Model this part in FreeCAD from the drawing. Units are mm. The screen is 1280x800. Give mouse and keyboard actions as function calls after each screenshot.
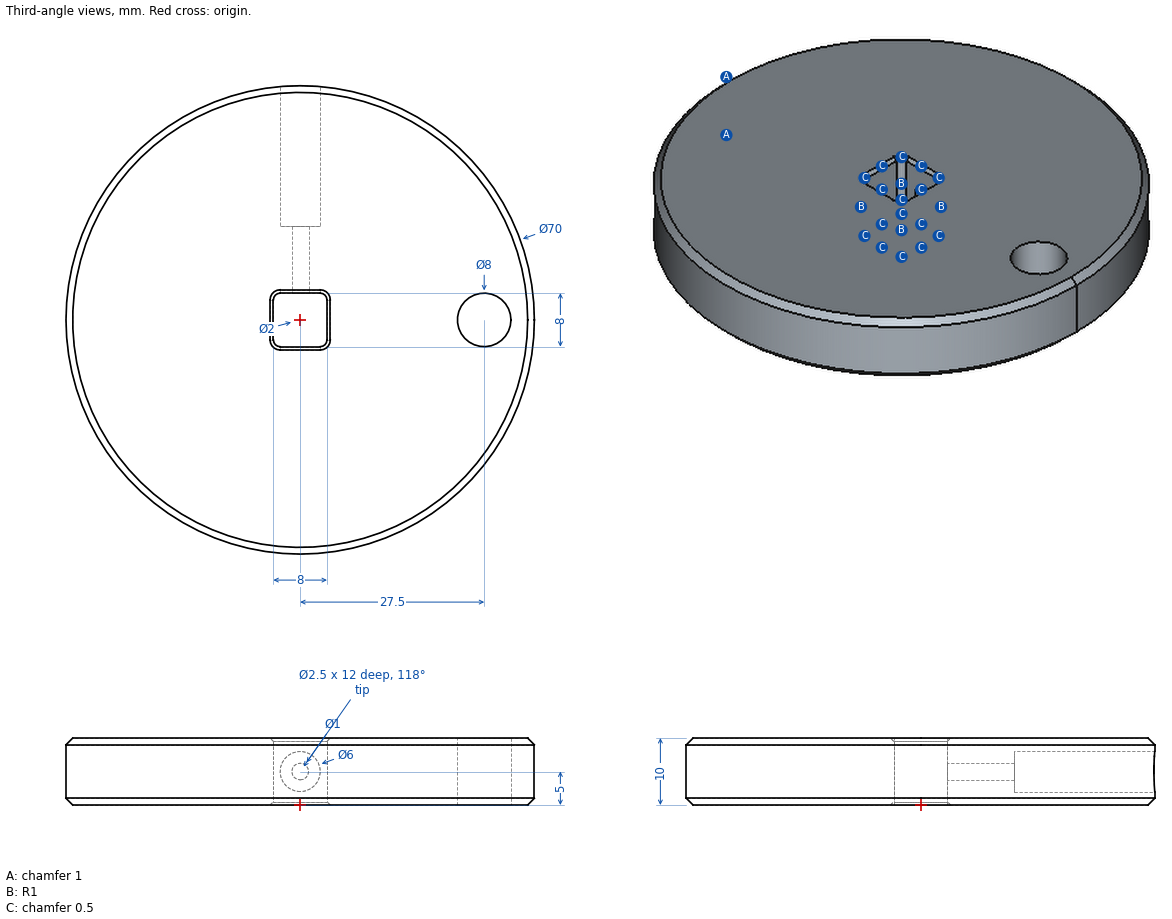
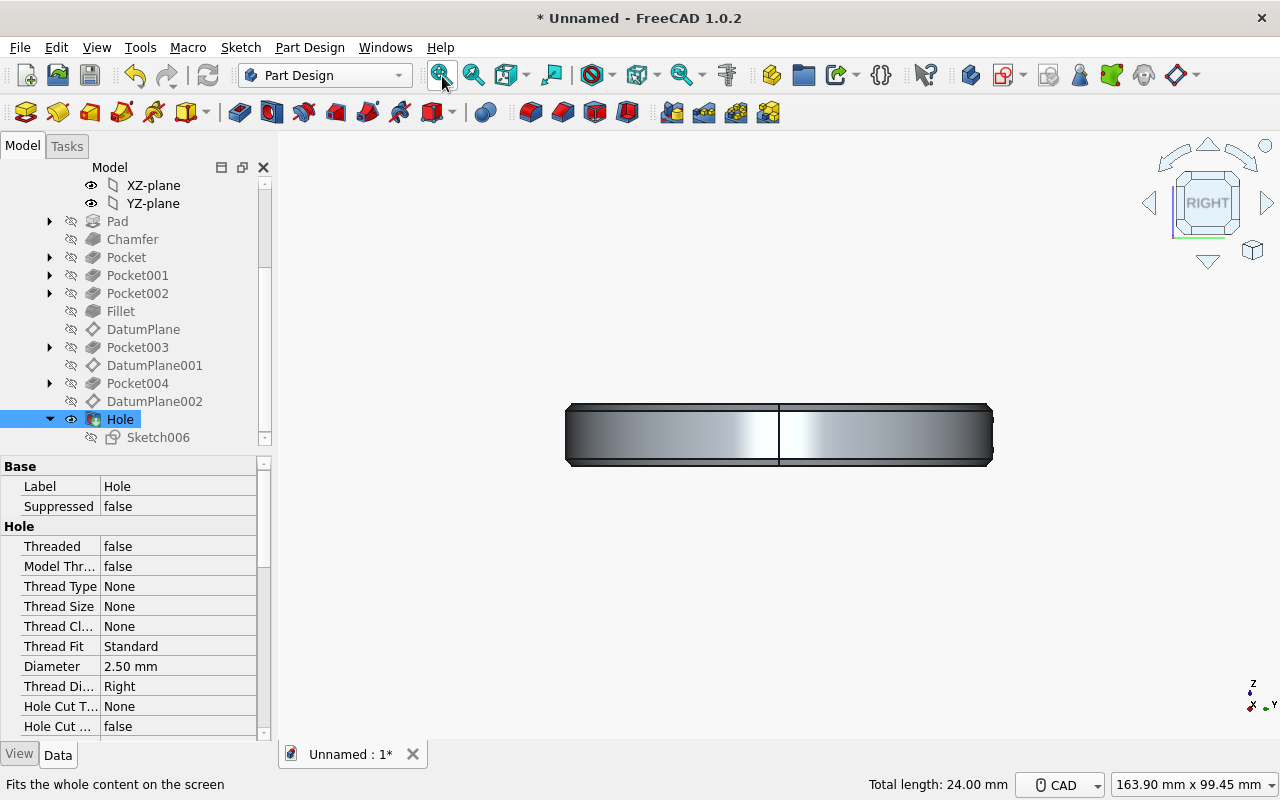
click(442, 76)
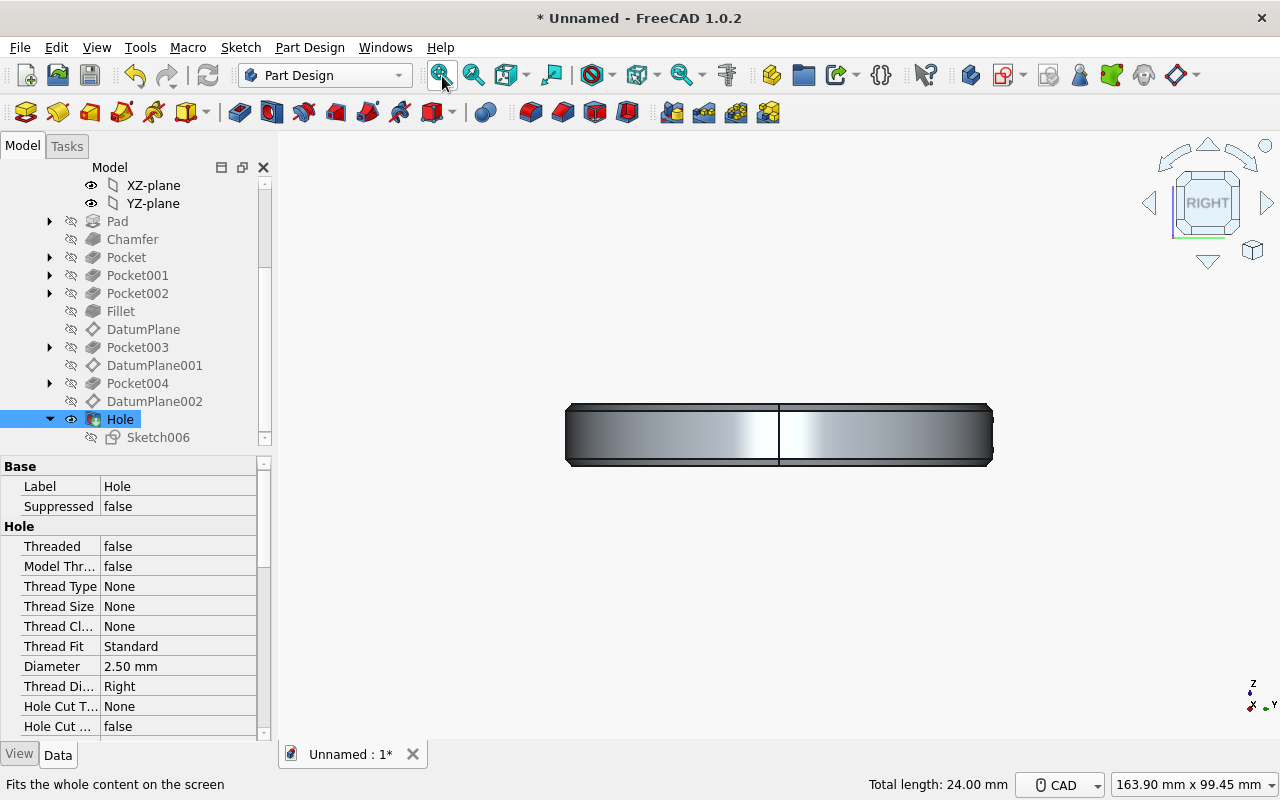
key(5)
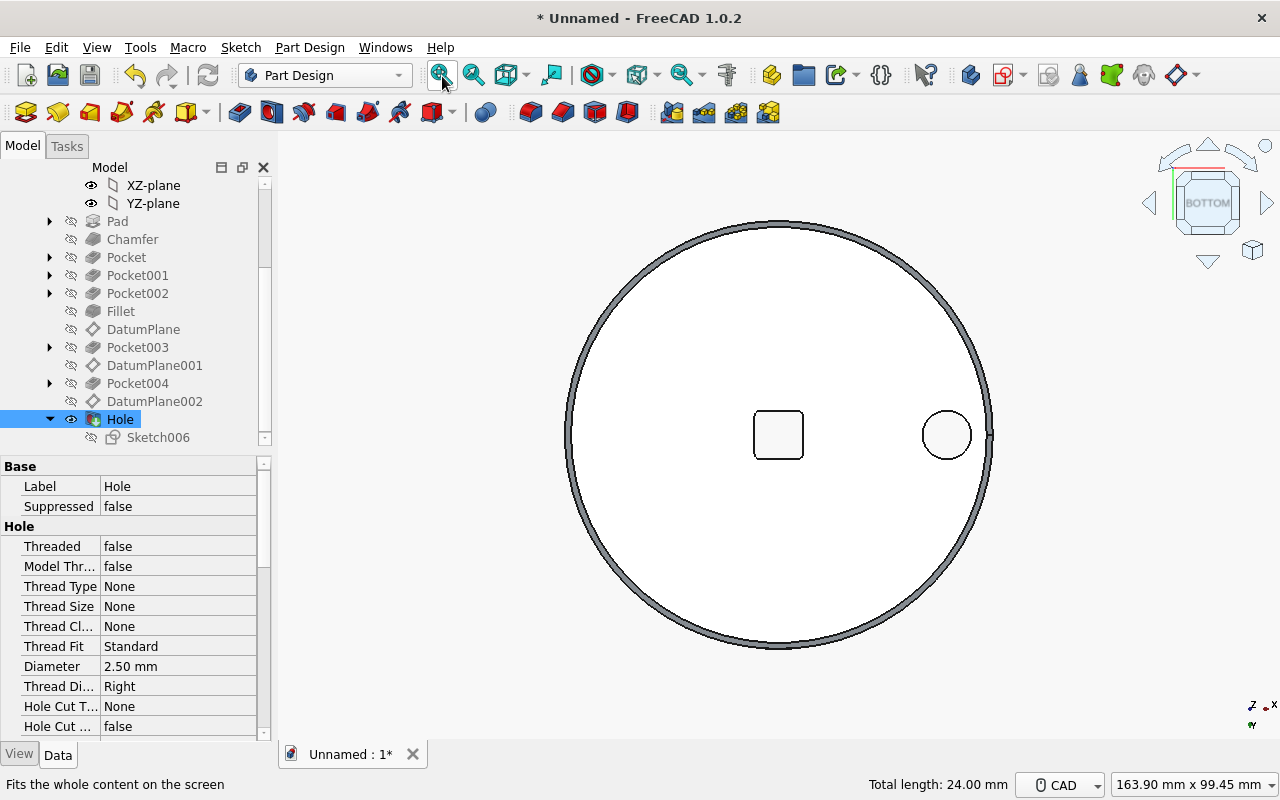
click(779, 410, ctrl)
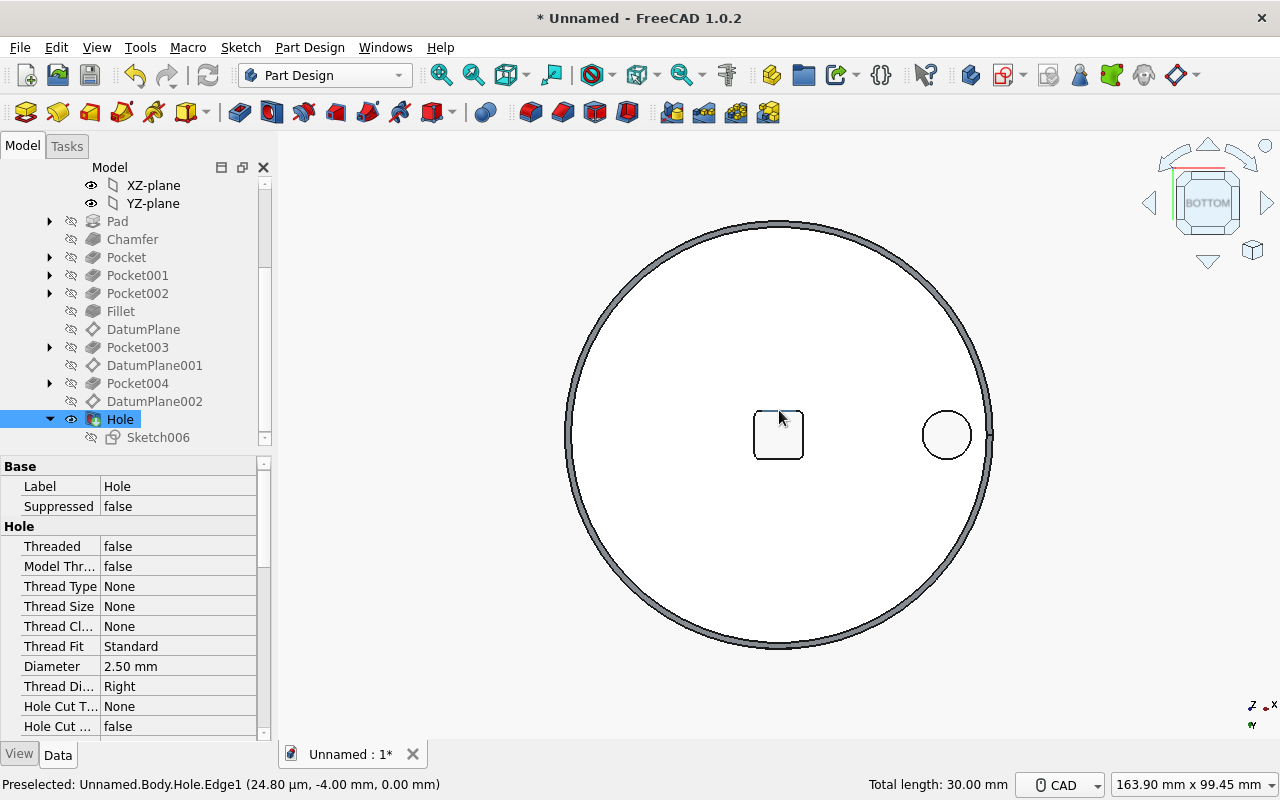
click(754, 434, ctrl)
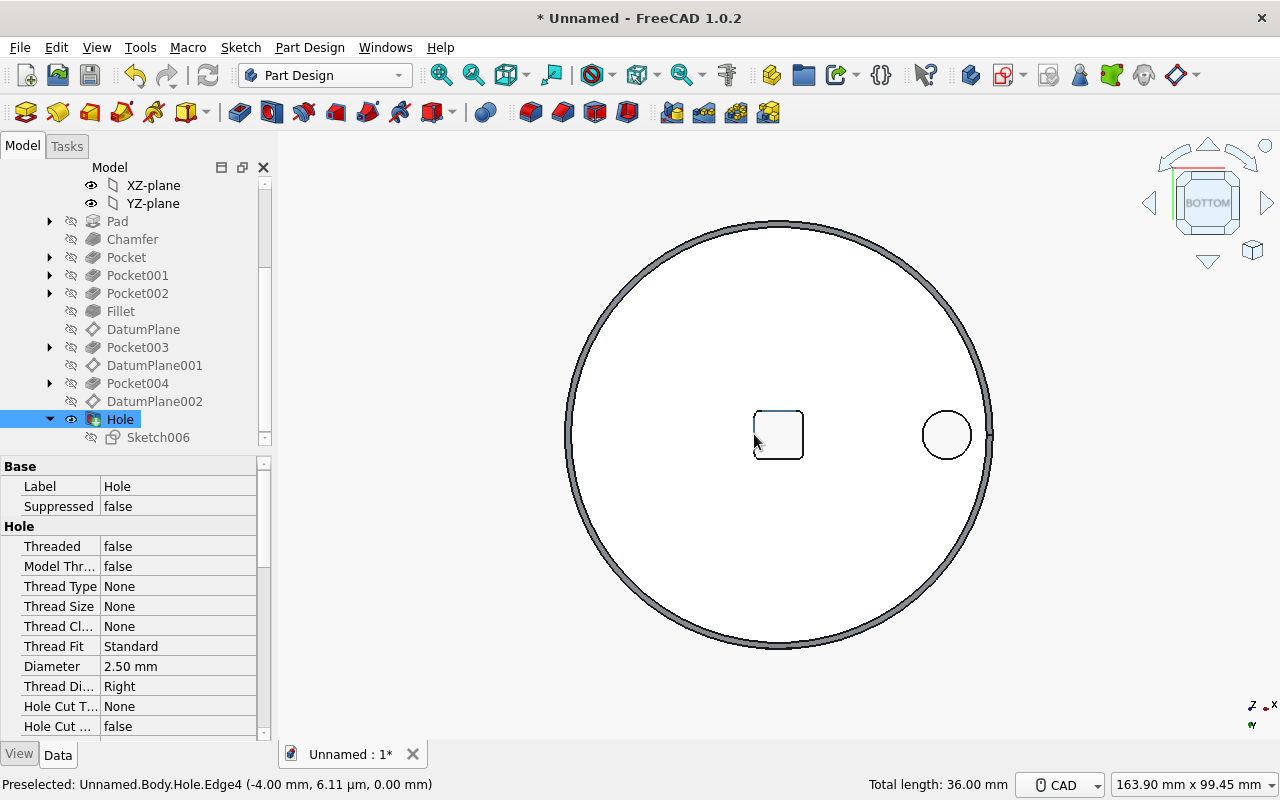
click(803, 434, ctrl)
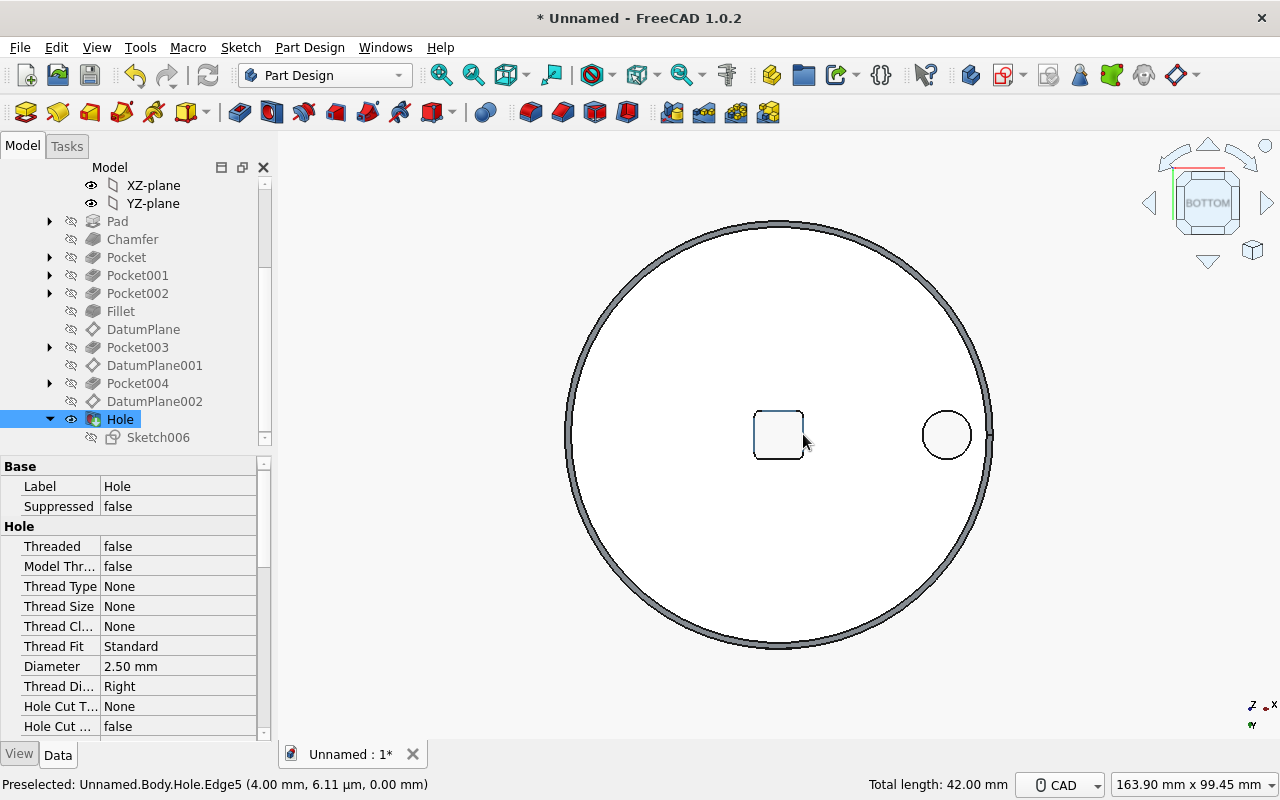
click(779, 458, ctrl)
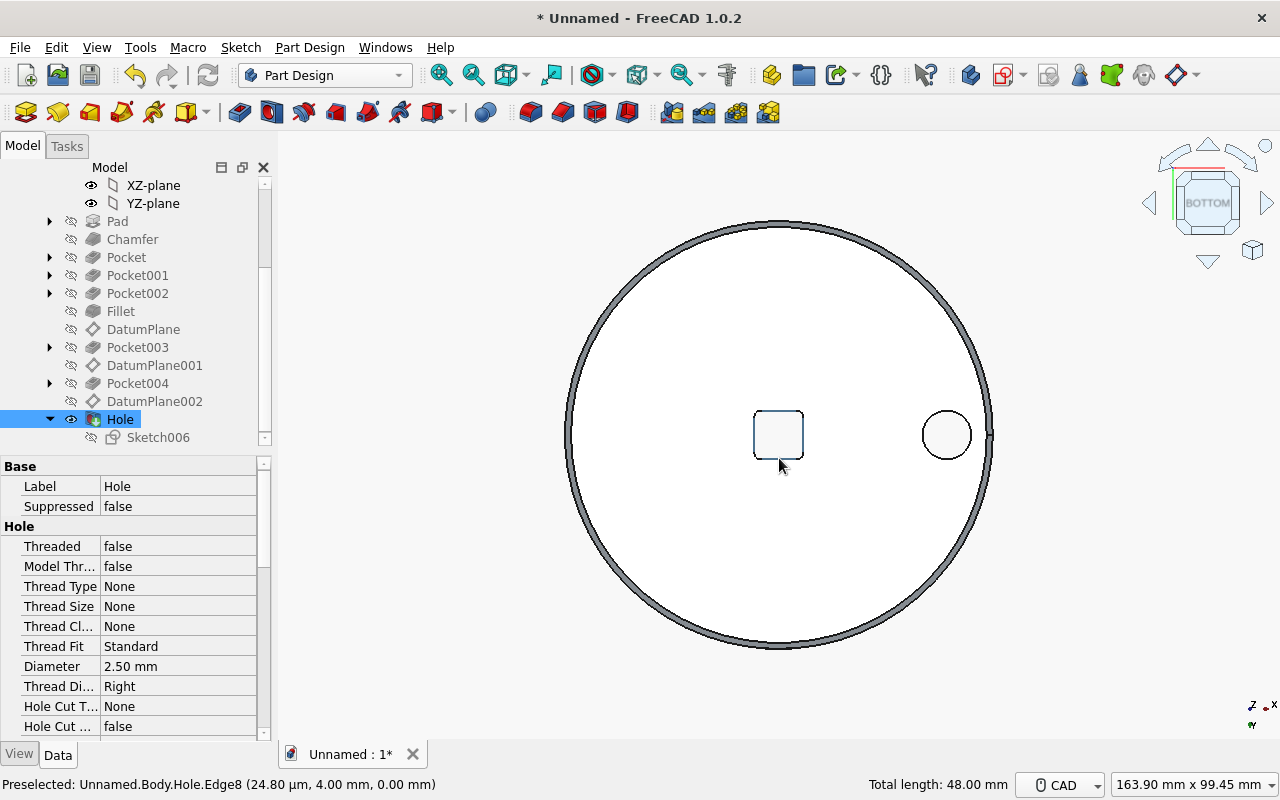
scroll(756, 411, up, 8)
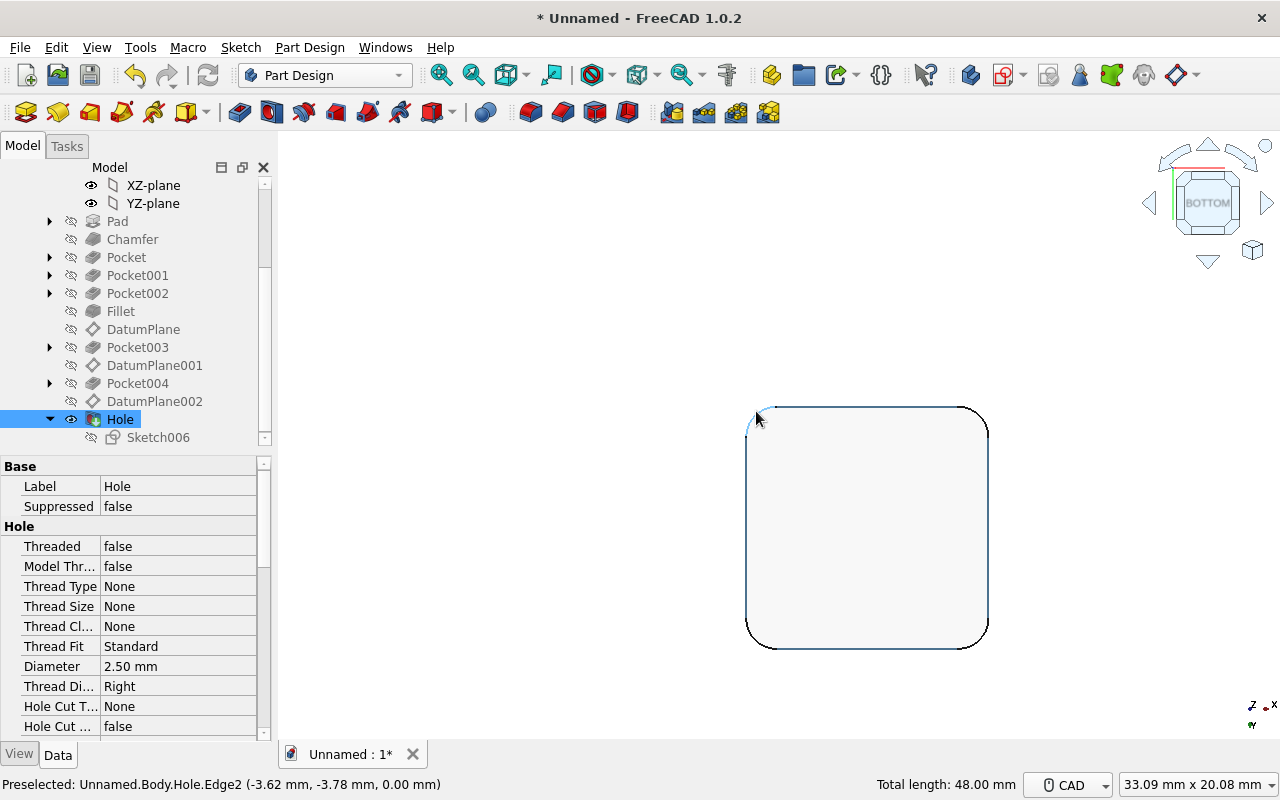
click(759, 412, ctrl)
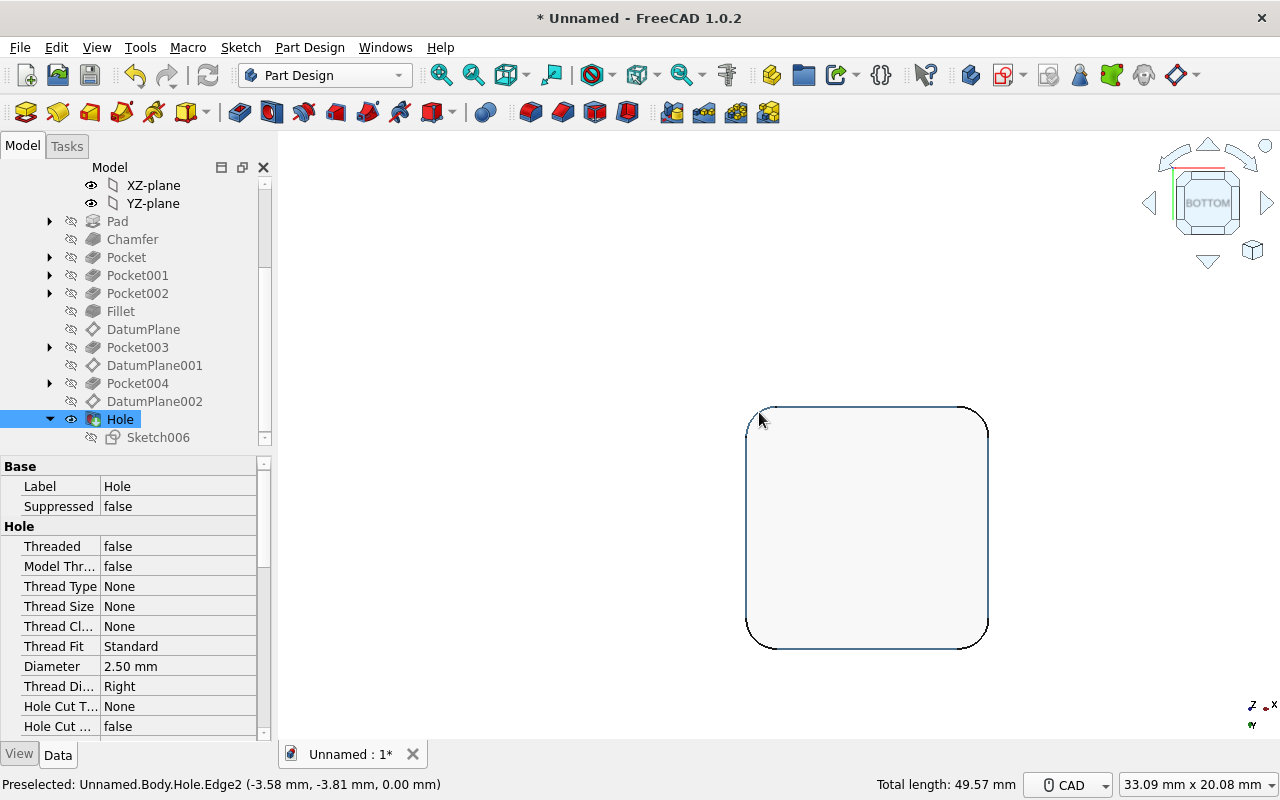
click(980, 415, ctrl)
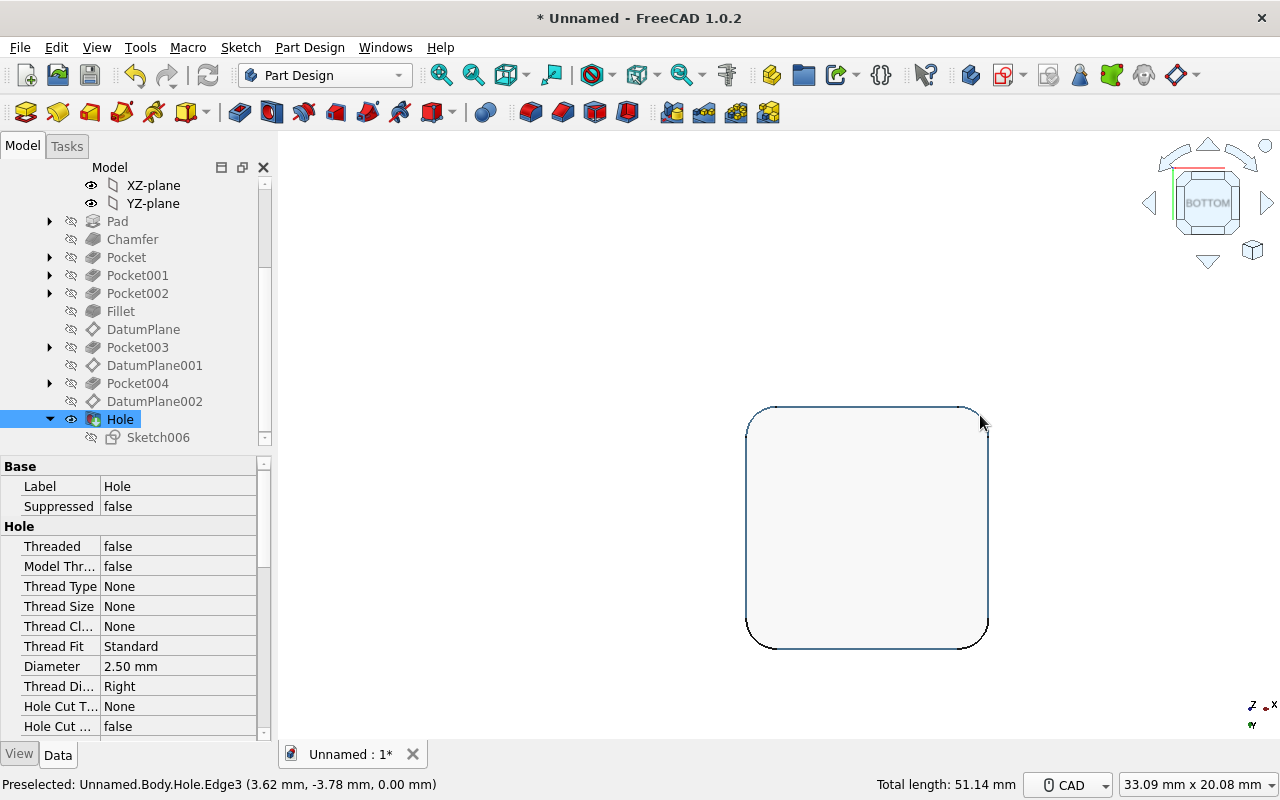
click(980, 639, ctrl)